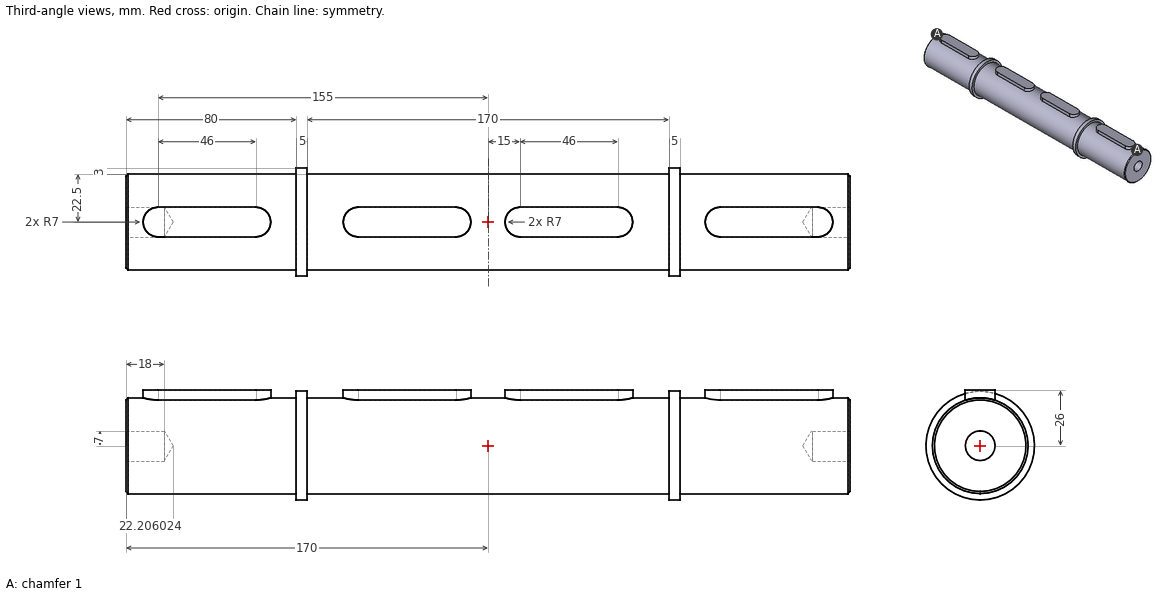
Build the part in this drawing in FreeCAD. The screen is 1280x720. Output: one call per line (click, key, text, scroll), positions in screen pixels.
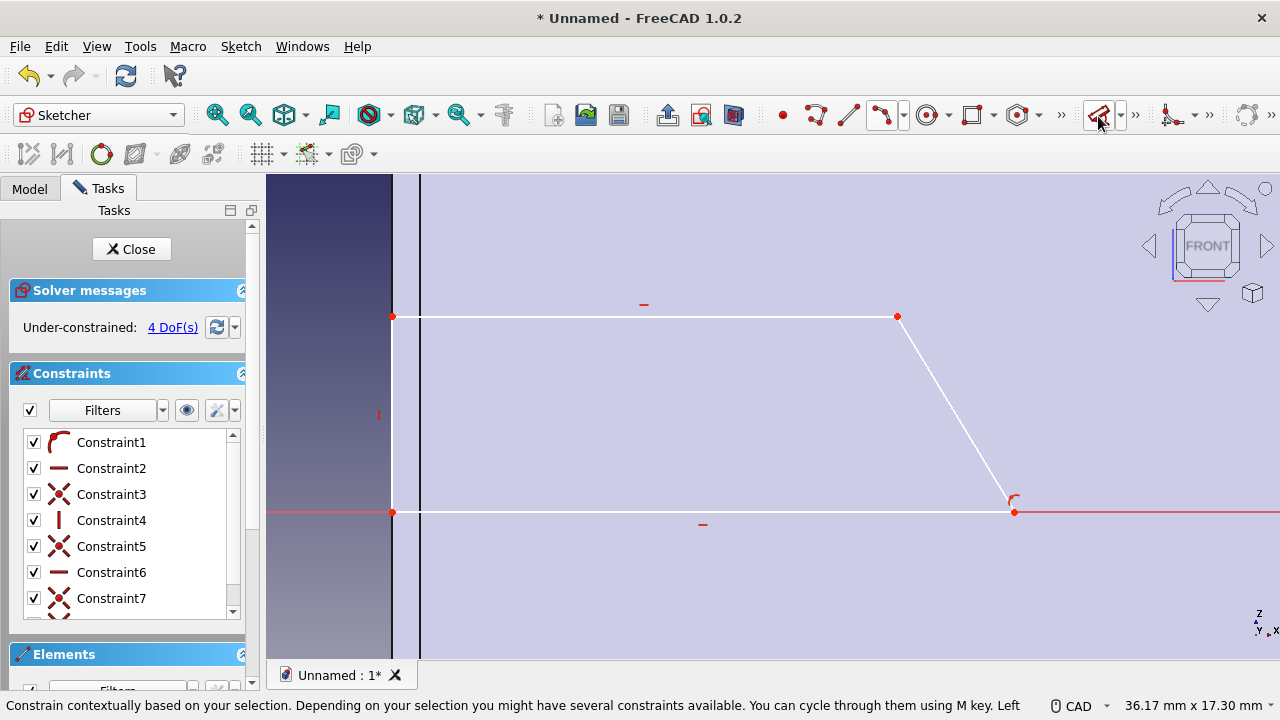
click(392, 454)
click(358, 415)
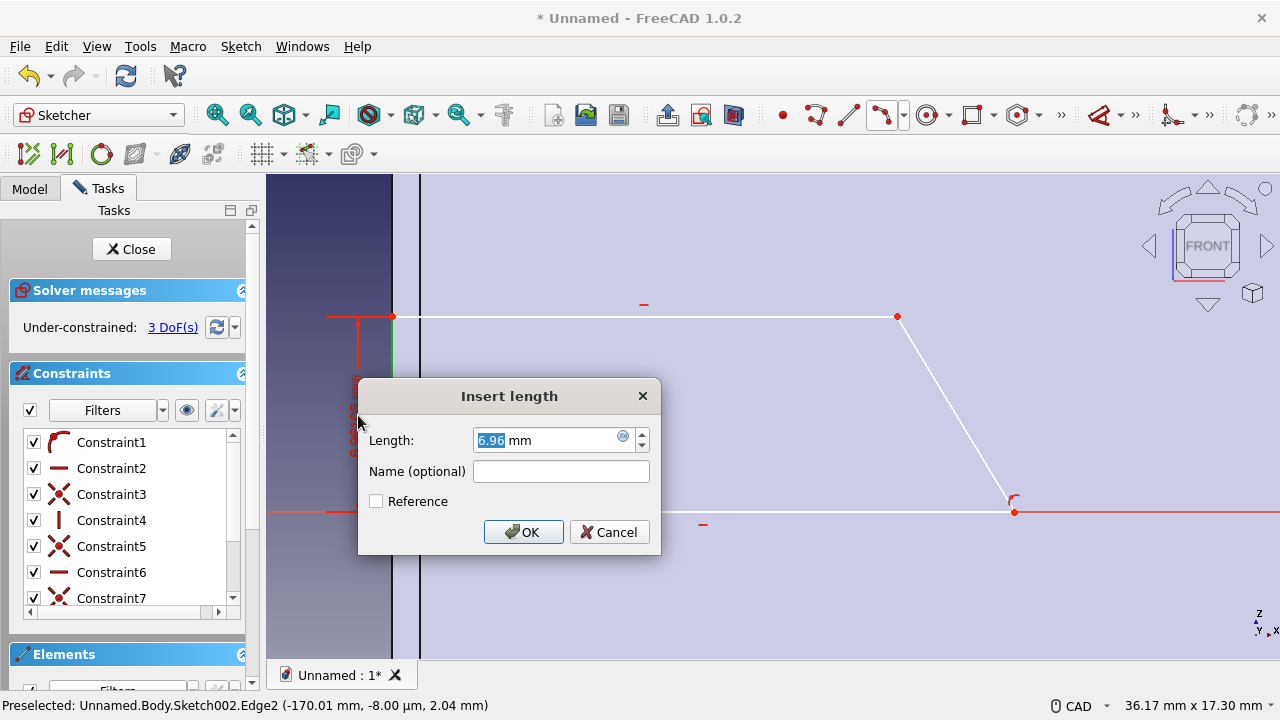
text(7)
key(Return)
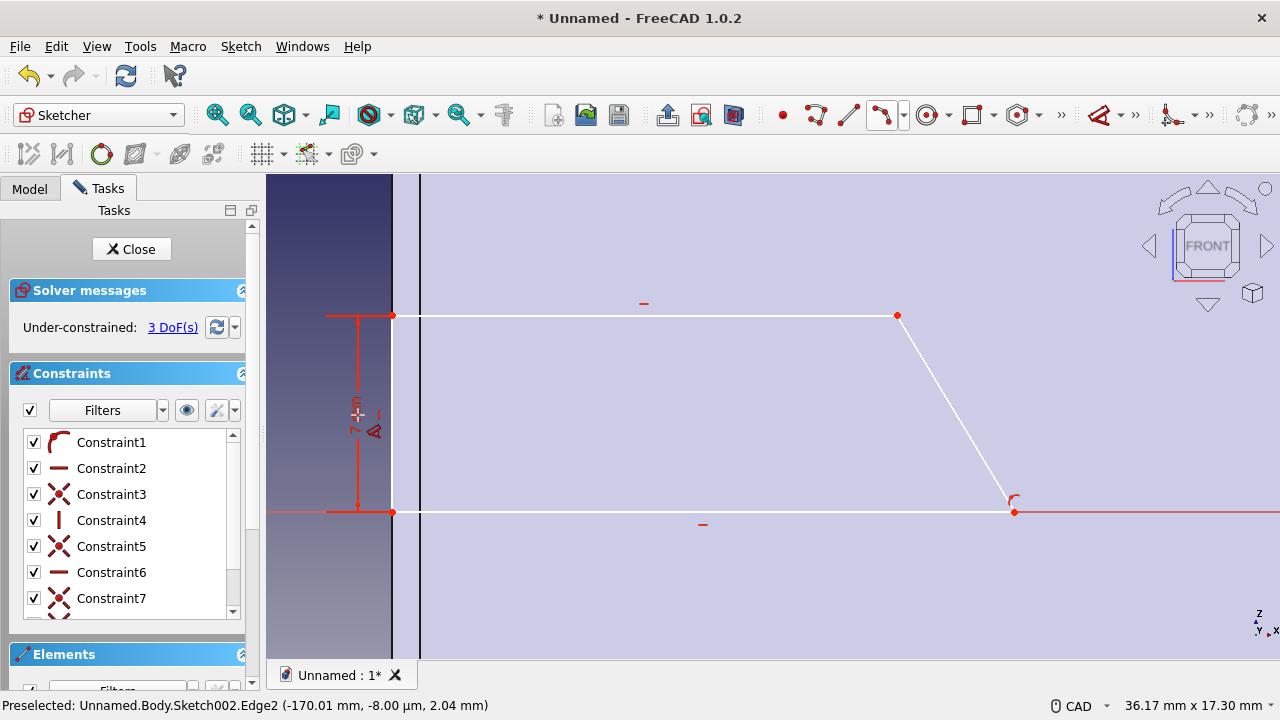
click(544, 316)
click(645, 282)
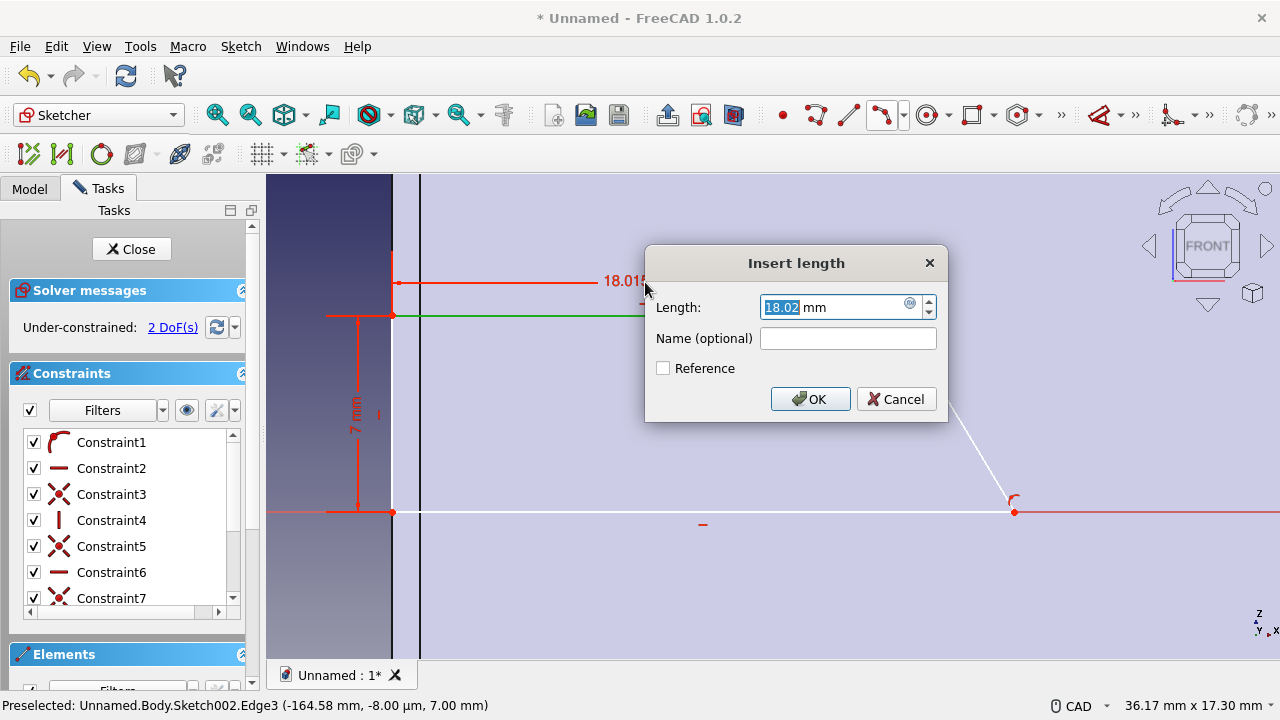
text(18)
key(Return)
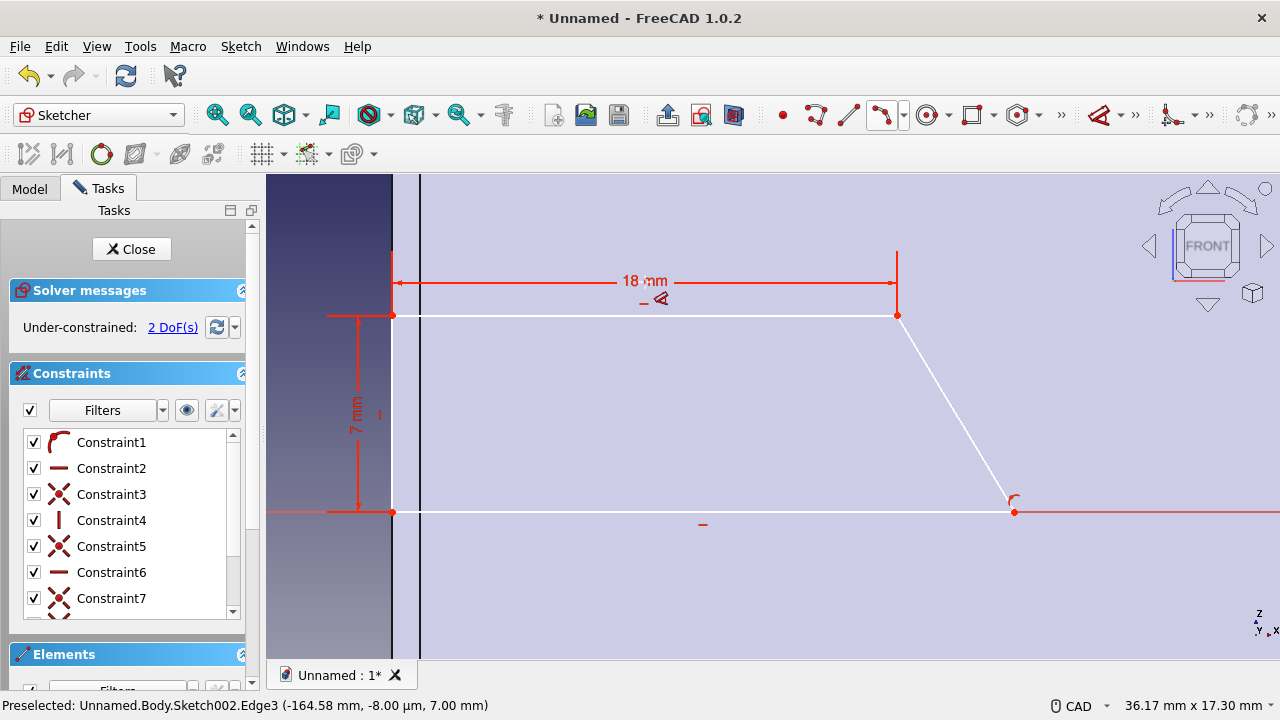
click(392, 512)
click(754, 546)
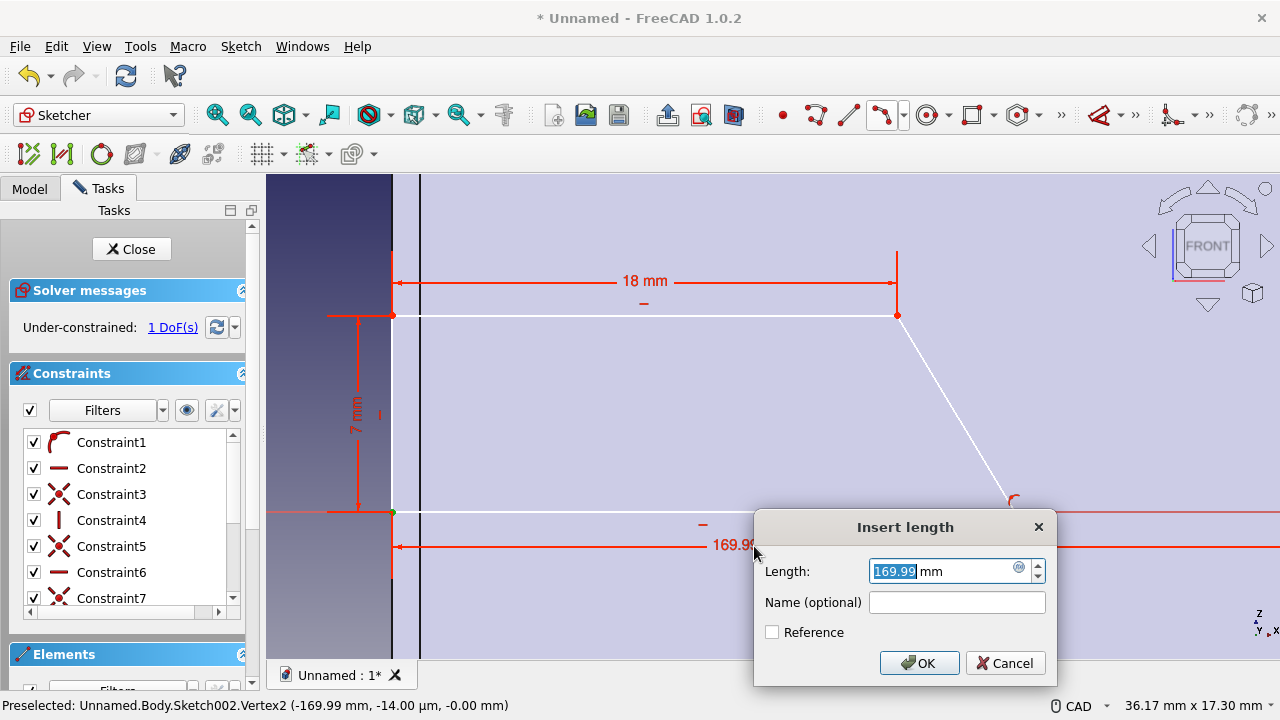
text(170)
key(Return)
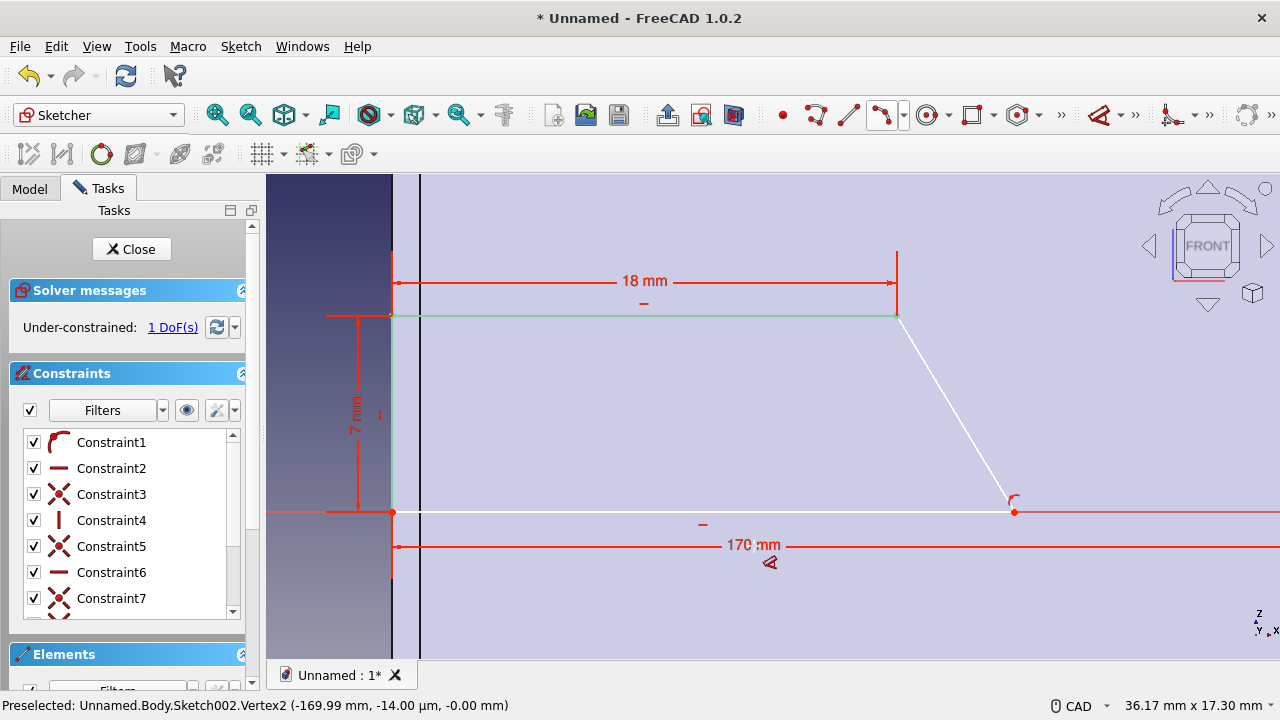
click(828, 512)
click(560, 546)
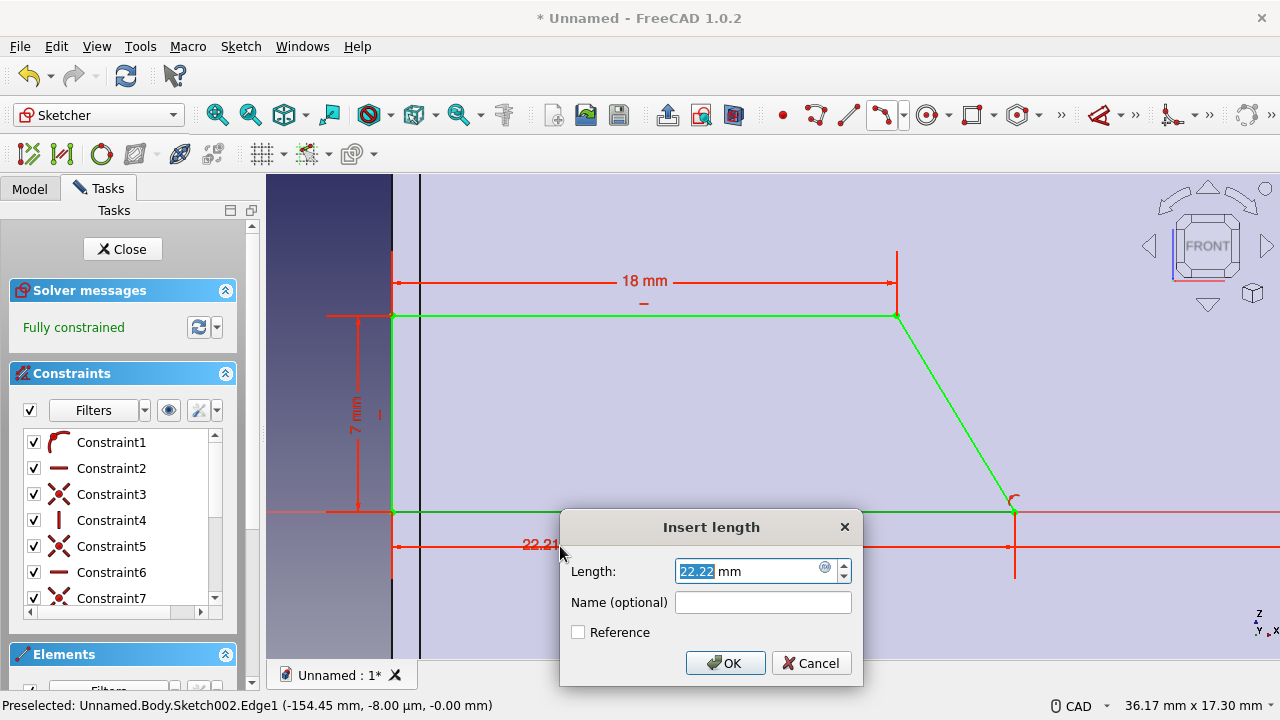
text(22.206024)
key(Return)
key(Escape)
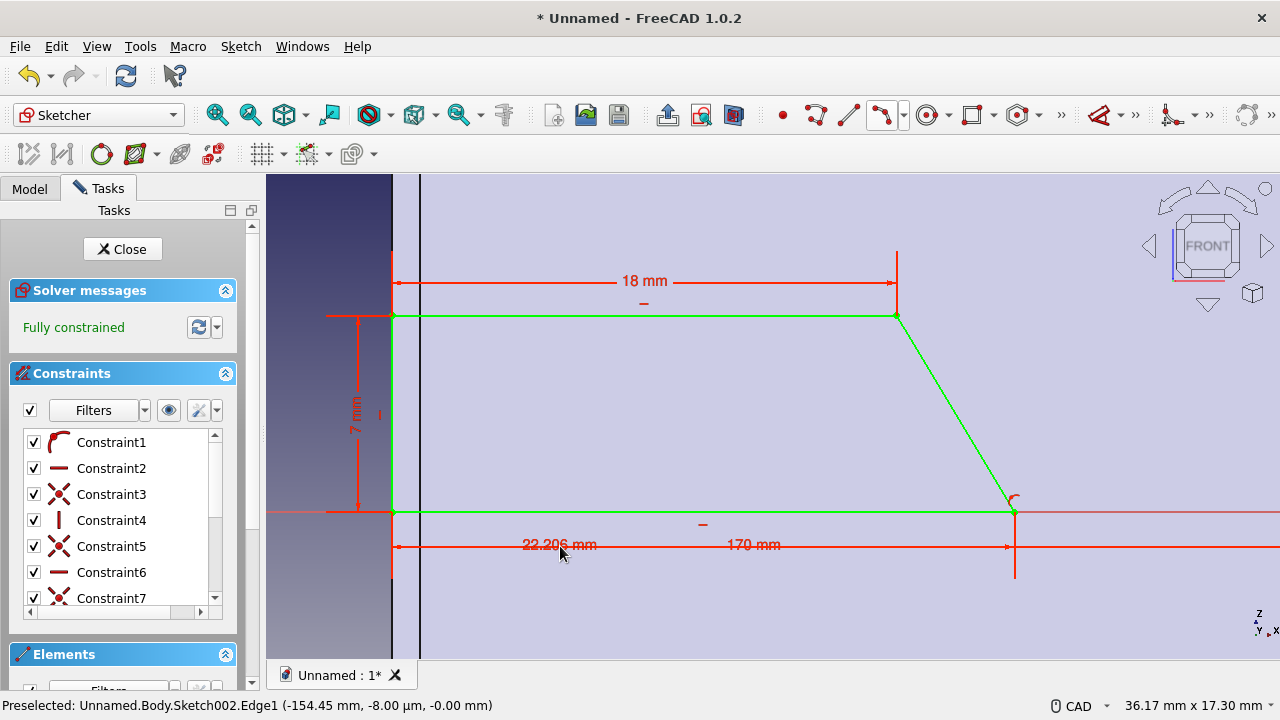
click(123, 249)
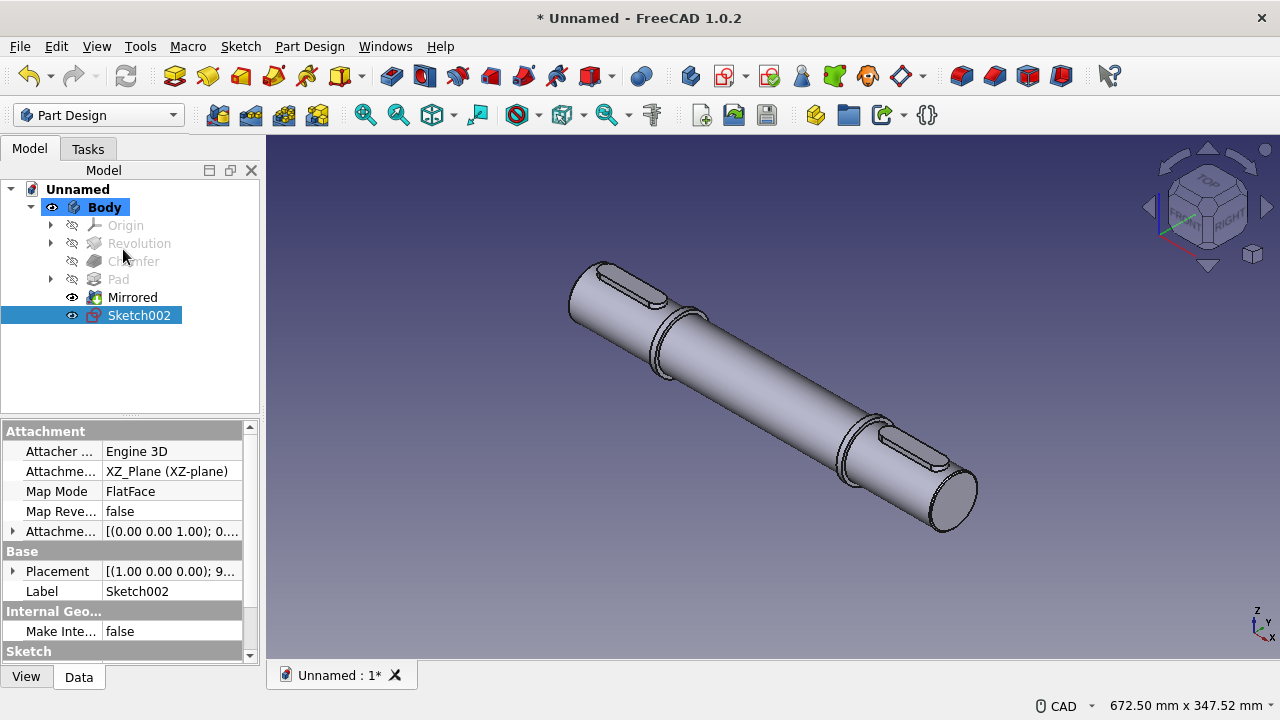
click(458, 76)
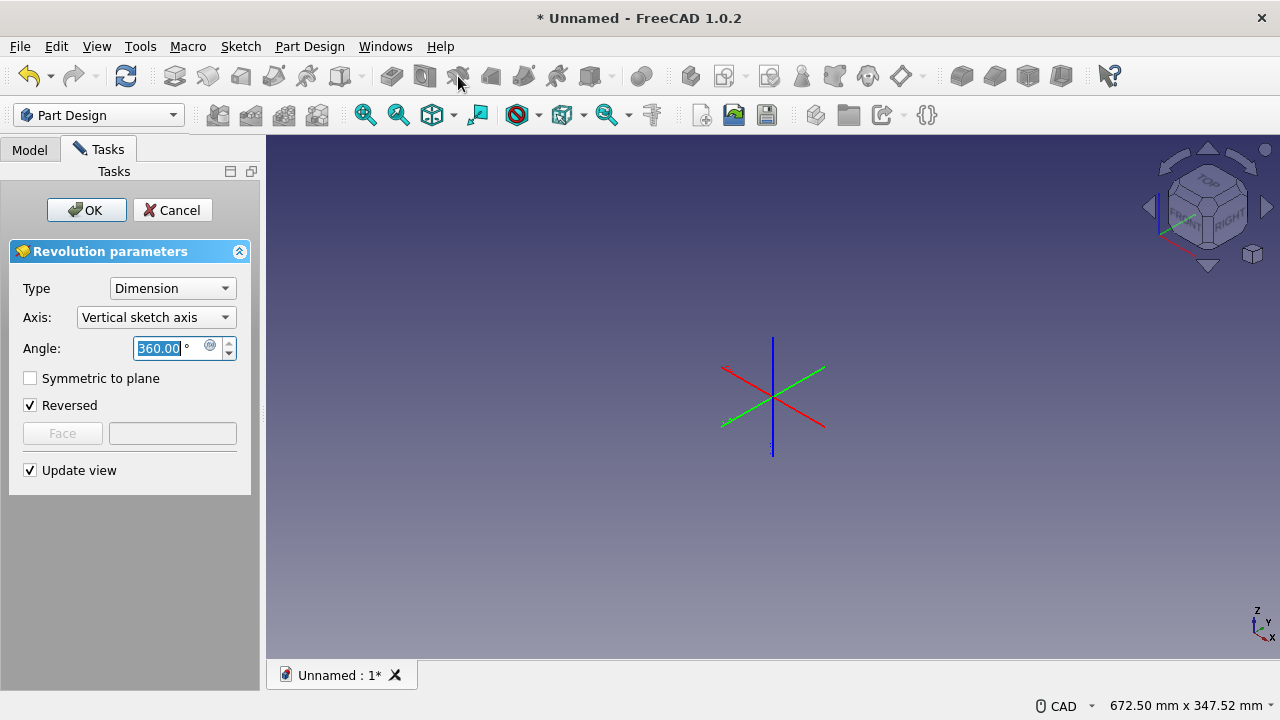
click(157, 318)